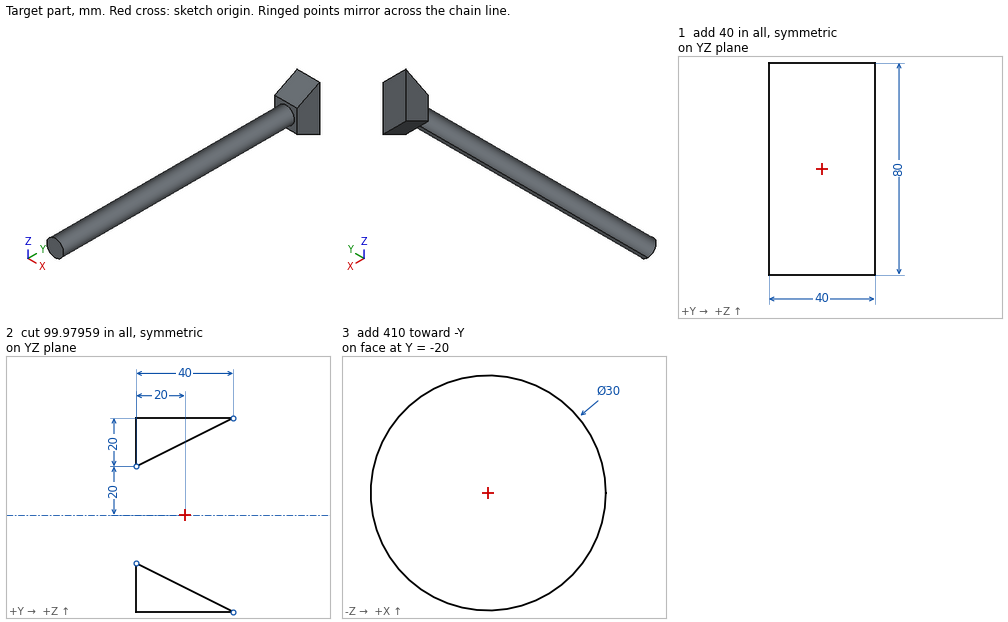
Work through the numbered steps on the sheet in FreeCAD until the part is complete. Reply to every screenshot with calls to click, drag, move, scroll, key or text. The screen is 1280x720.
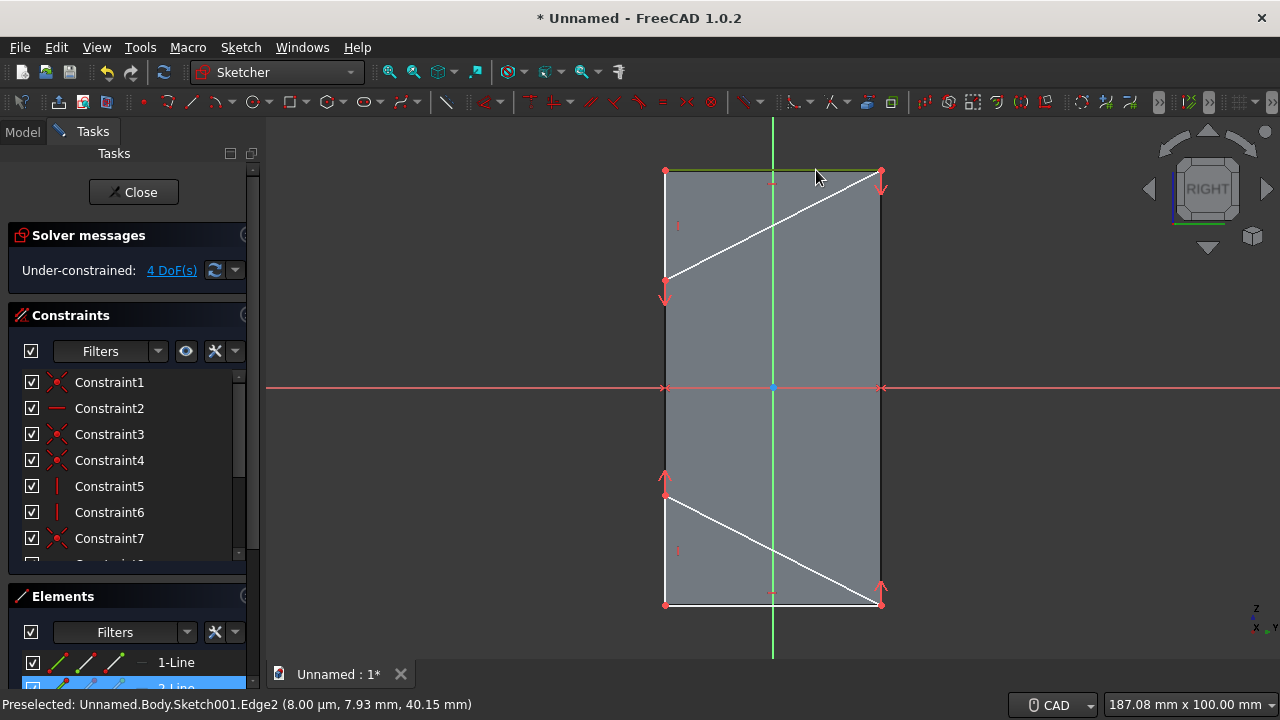
click(502, 102)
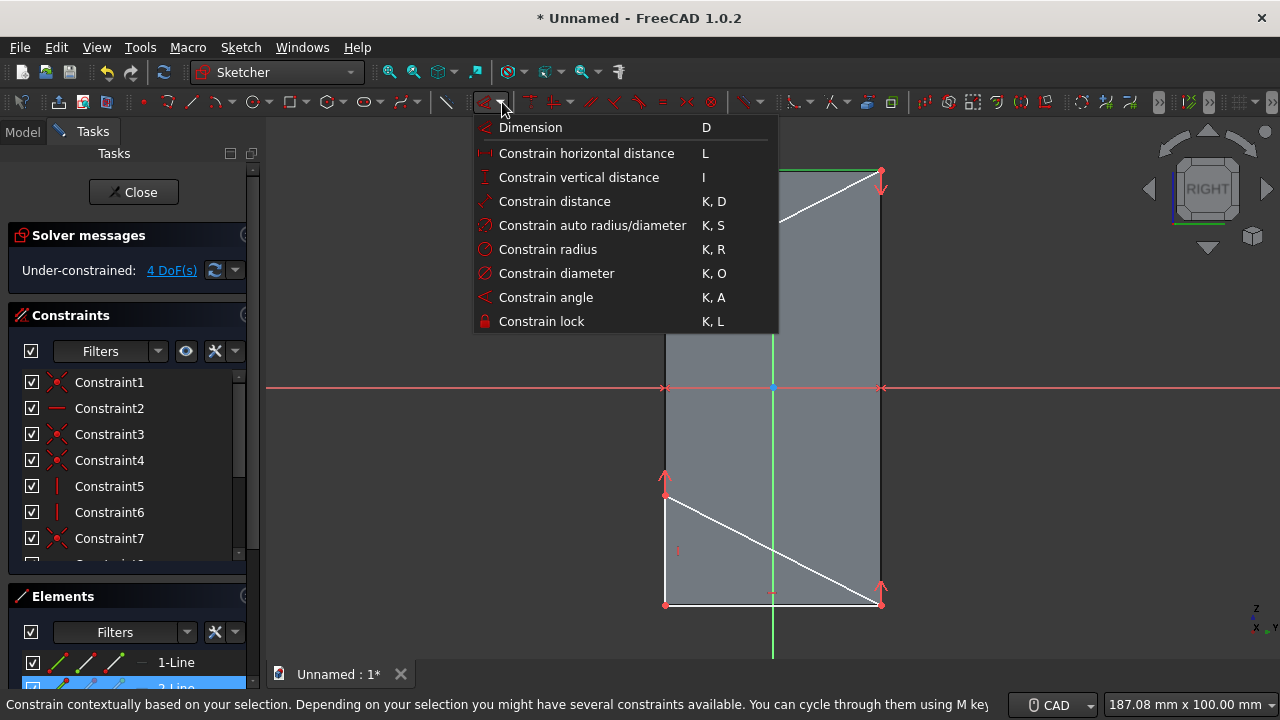
click(626, 153)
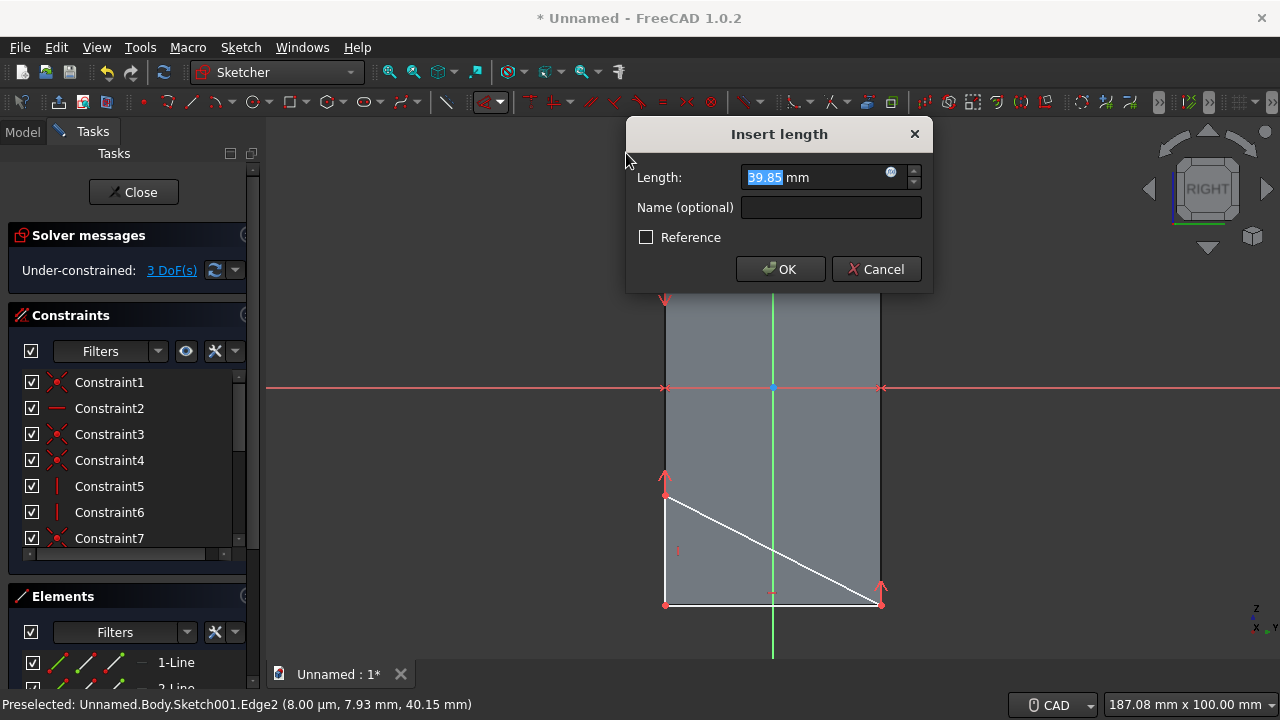
text(40)
key(Return)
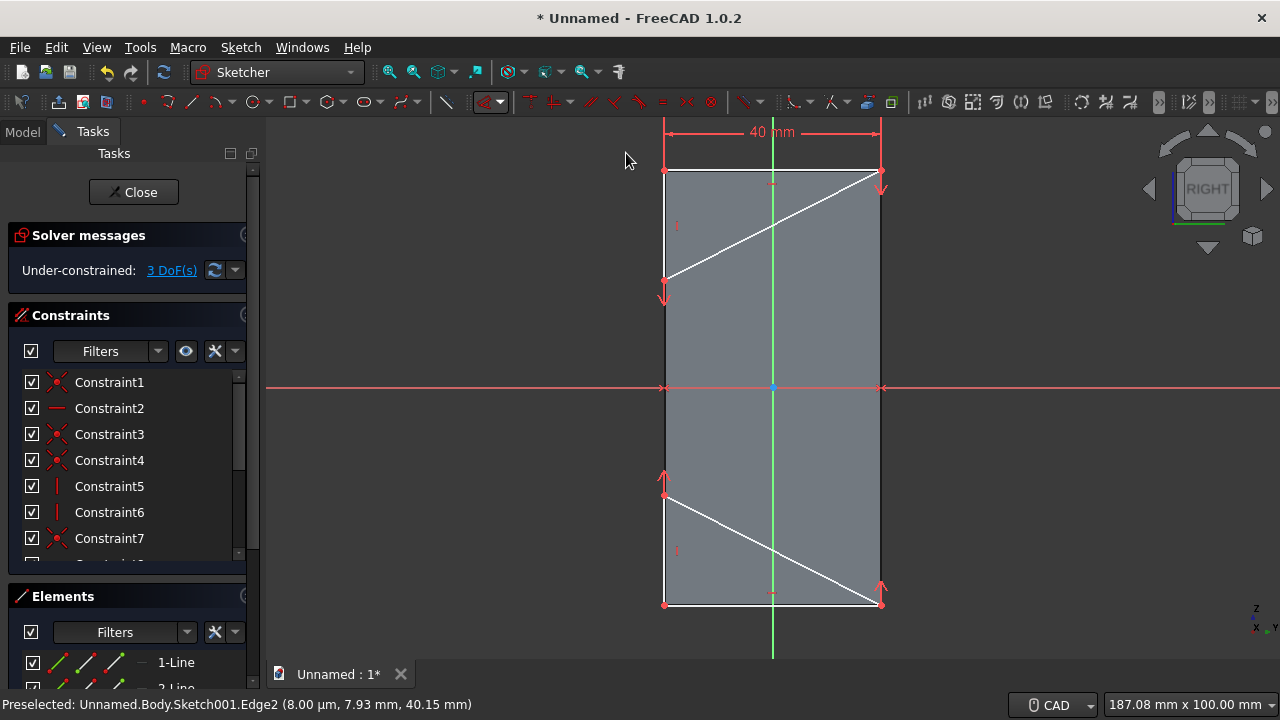
click(664, 203)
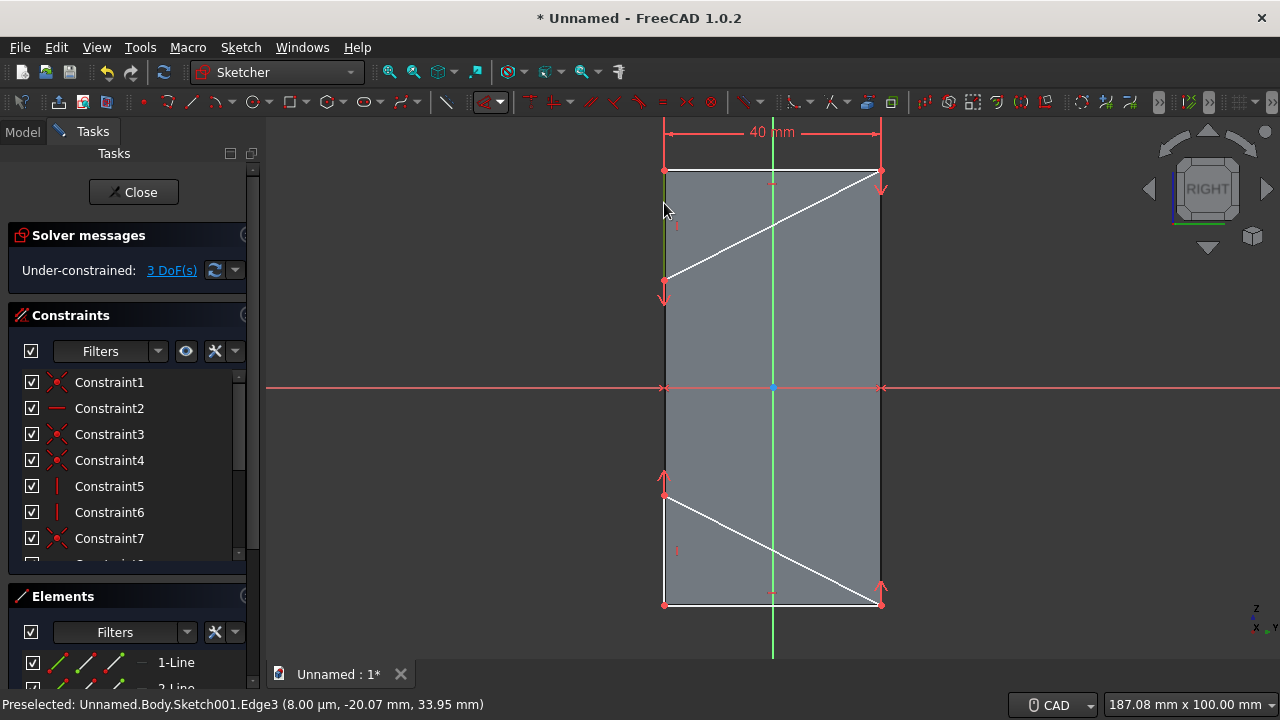
key(i)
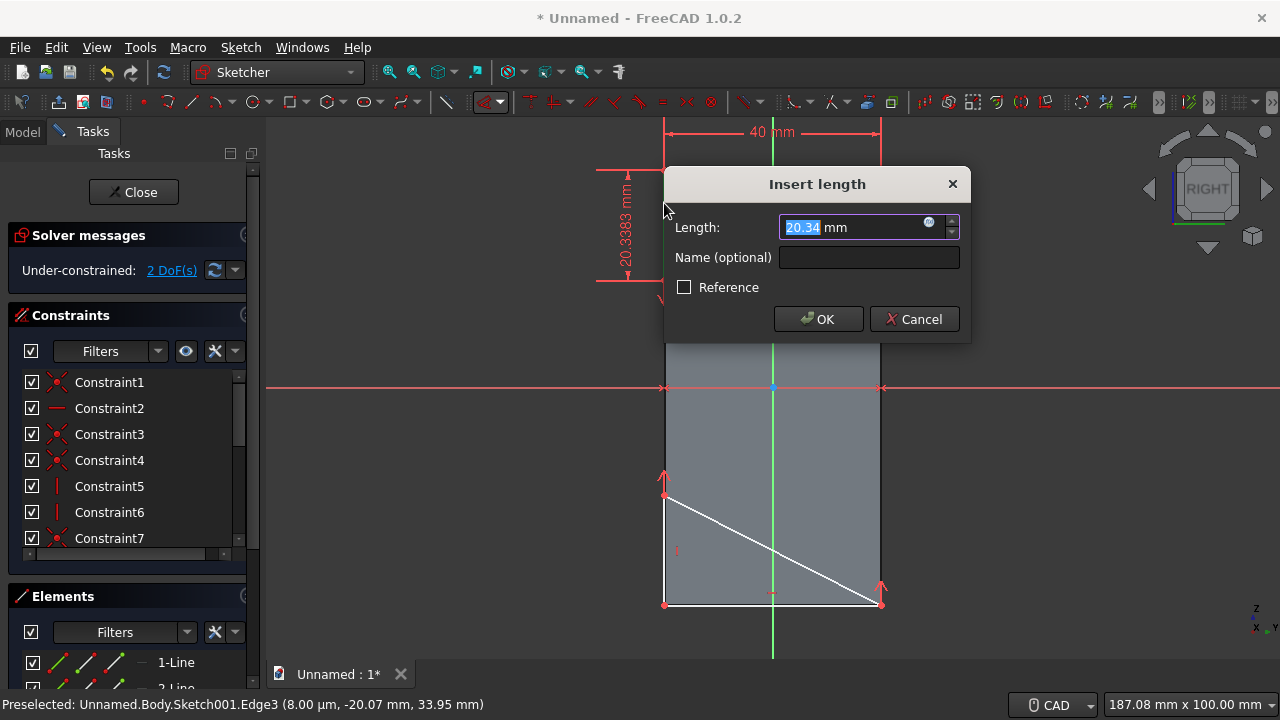
text(20)
key(Return)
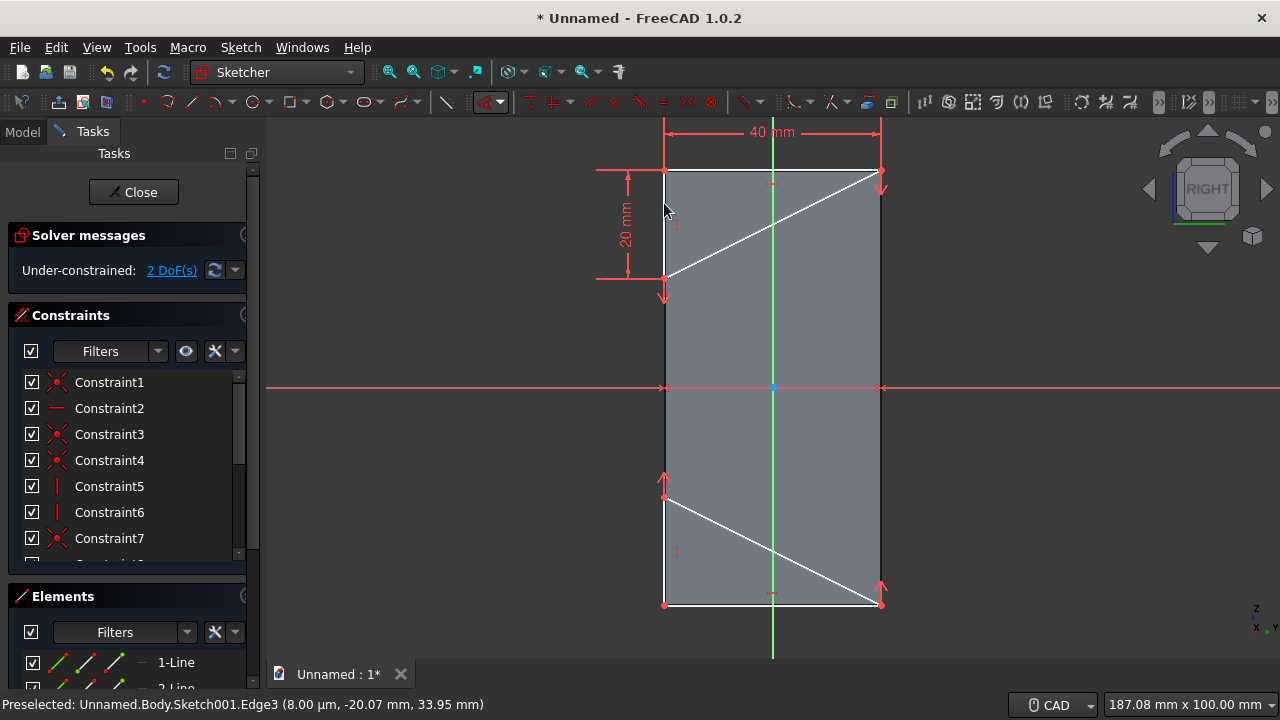
click(664, 279)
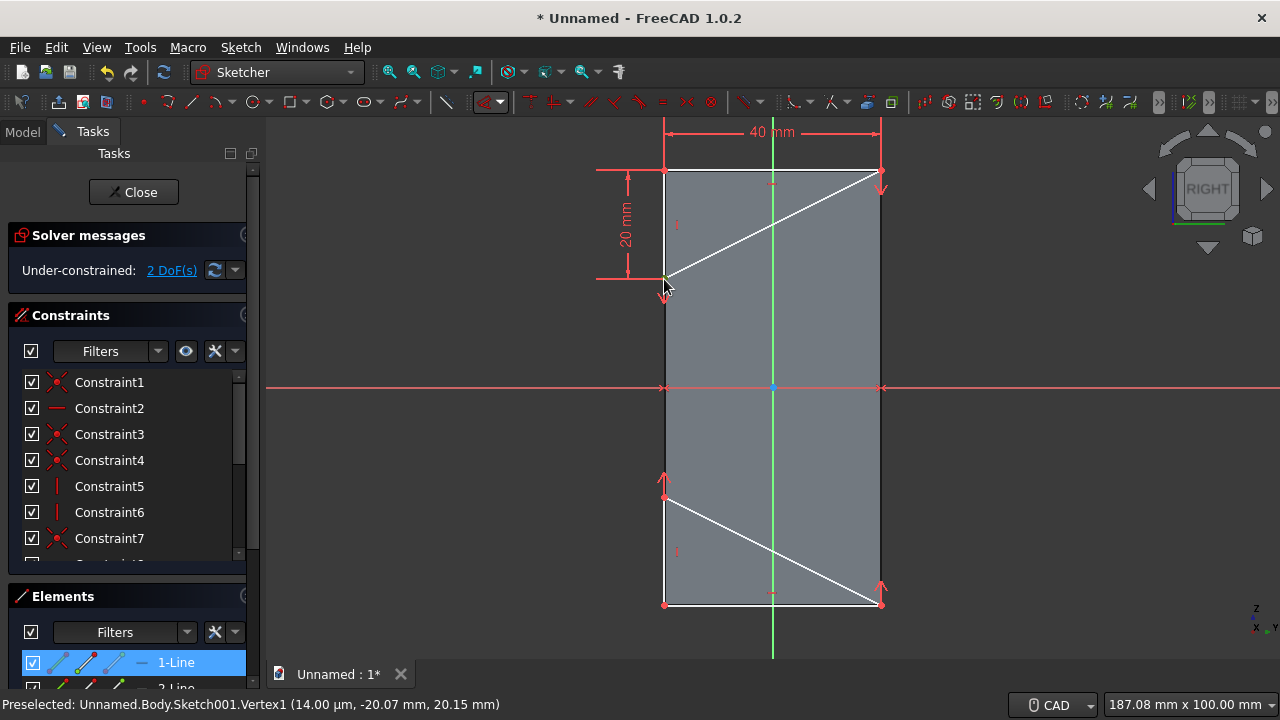
key(l)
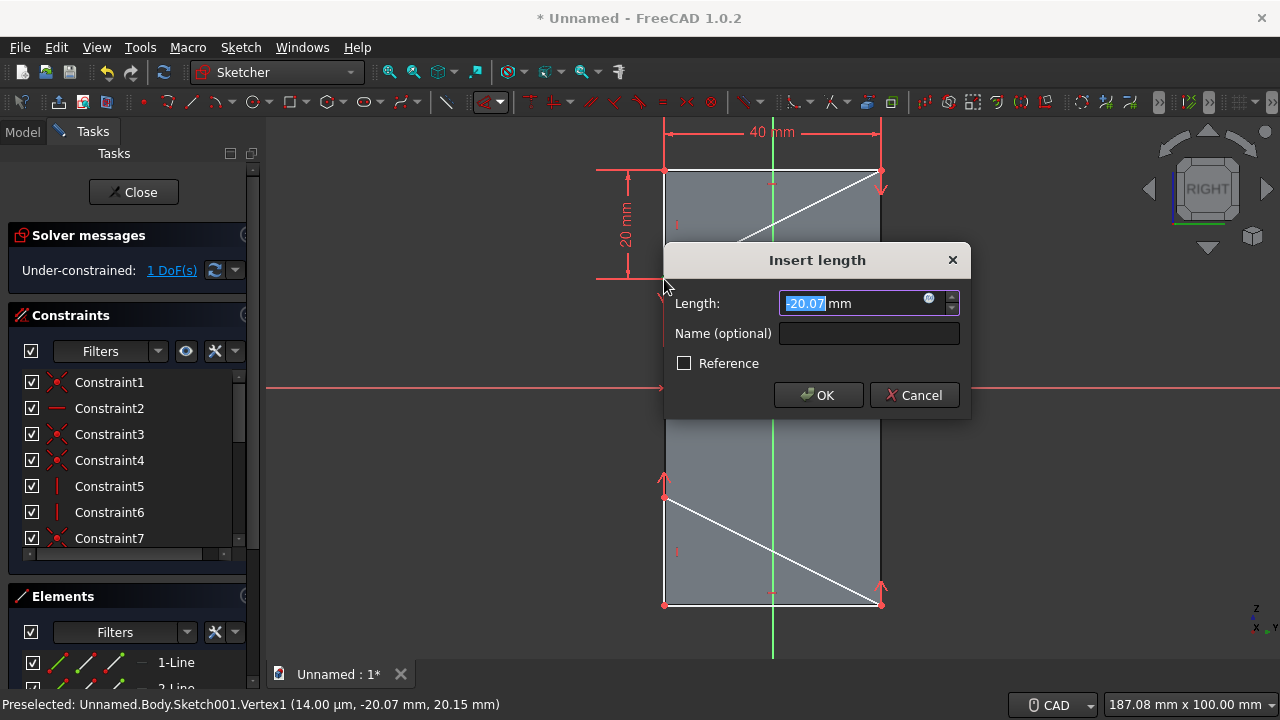
text(-20)
key(Return)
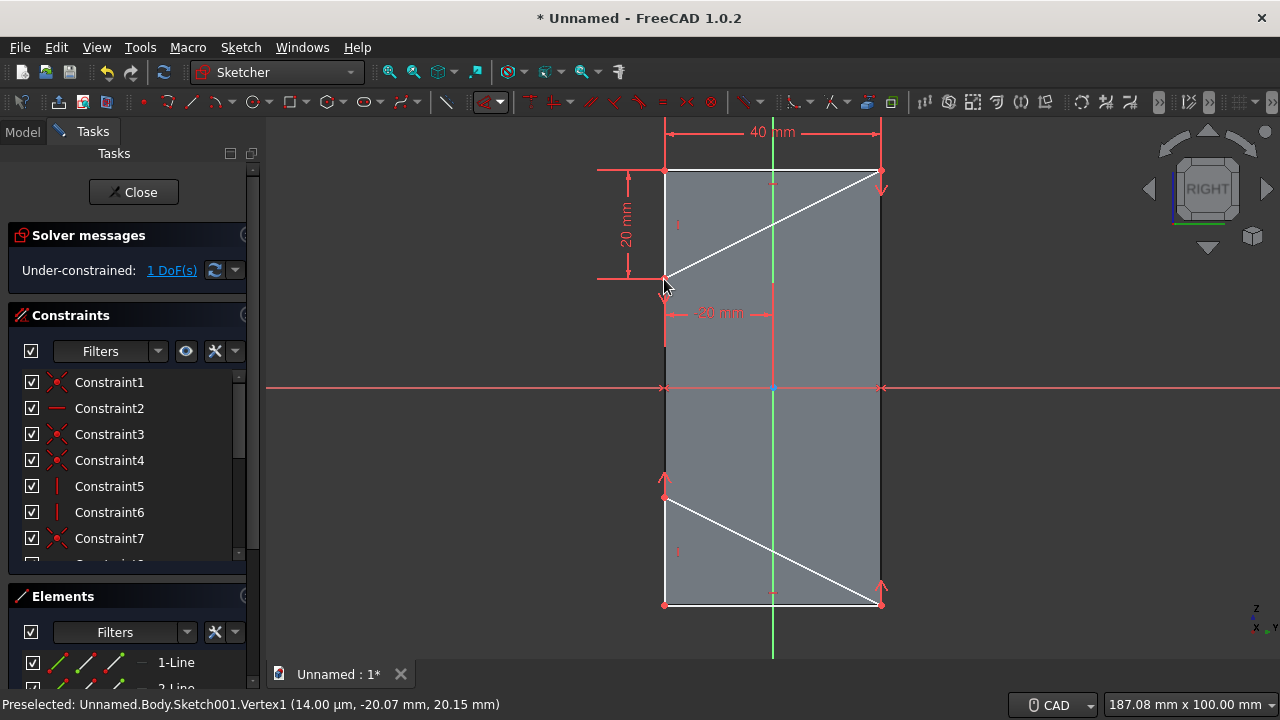
click(665, 279)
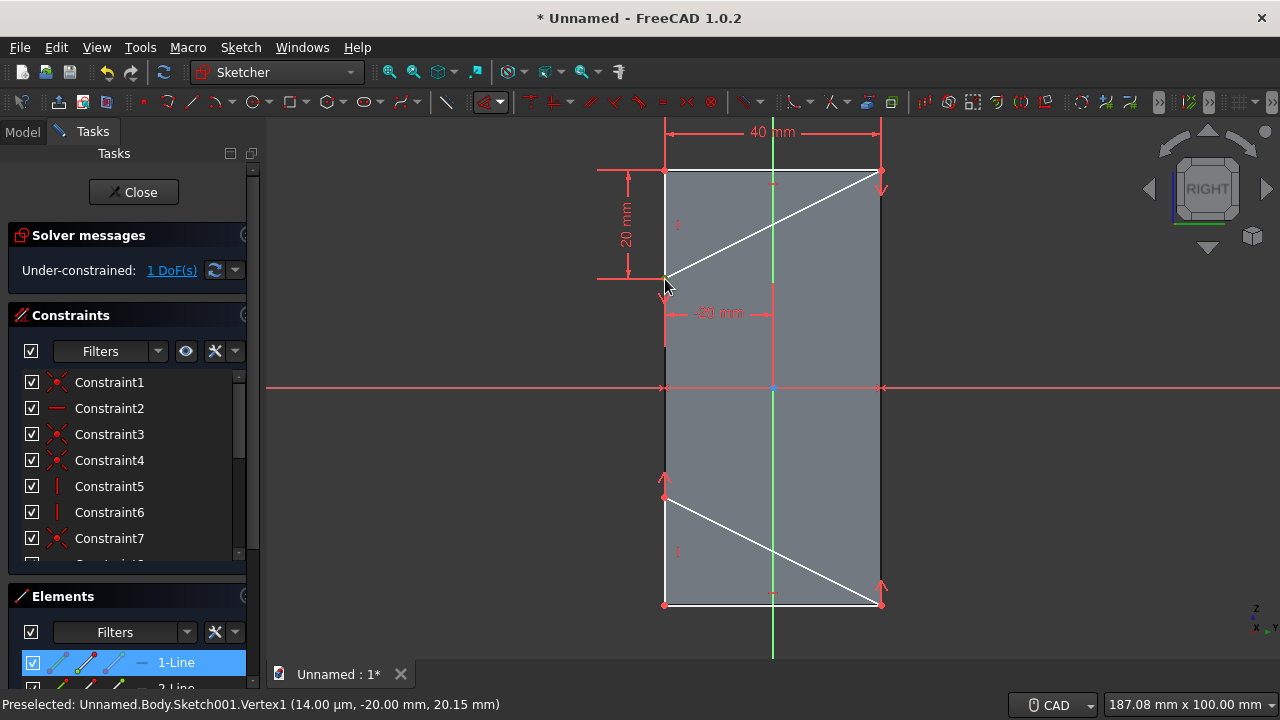
key(i)